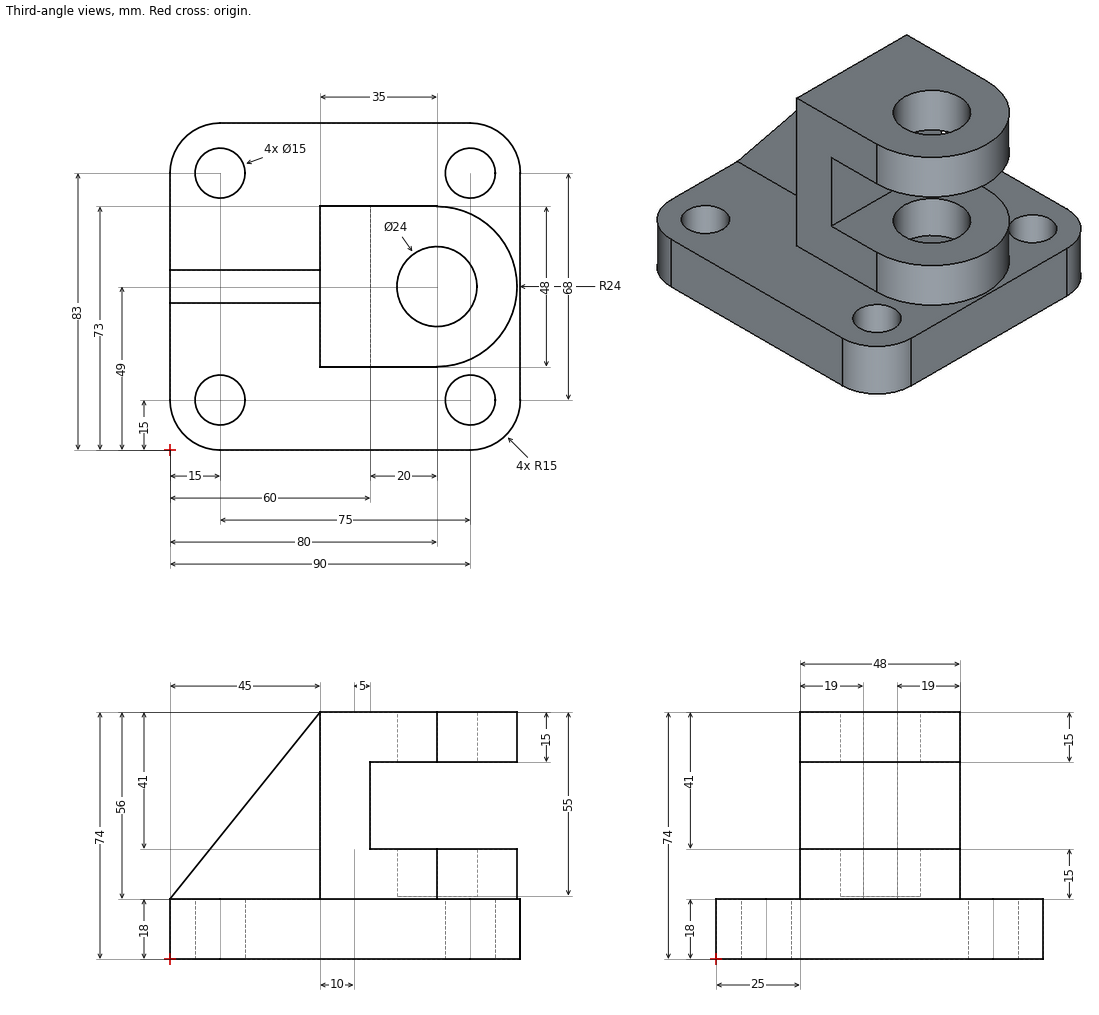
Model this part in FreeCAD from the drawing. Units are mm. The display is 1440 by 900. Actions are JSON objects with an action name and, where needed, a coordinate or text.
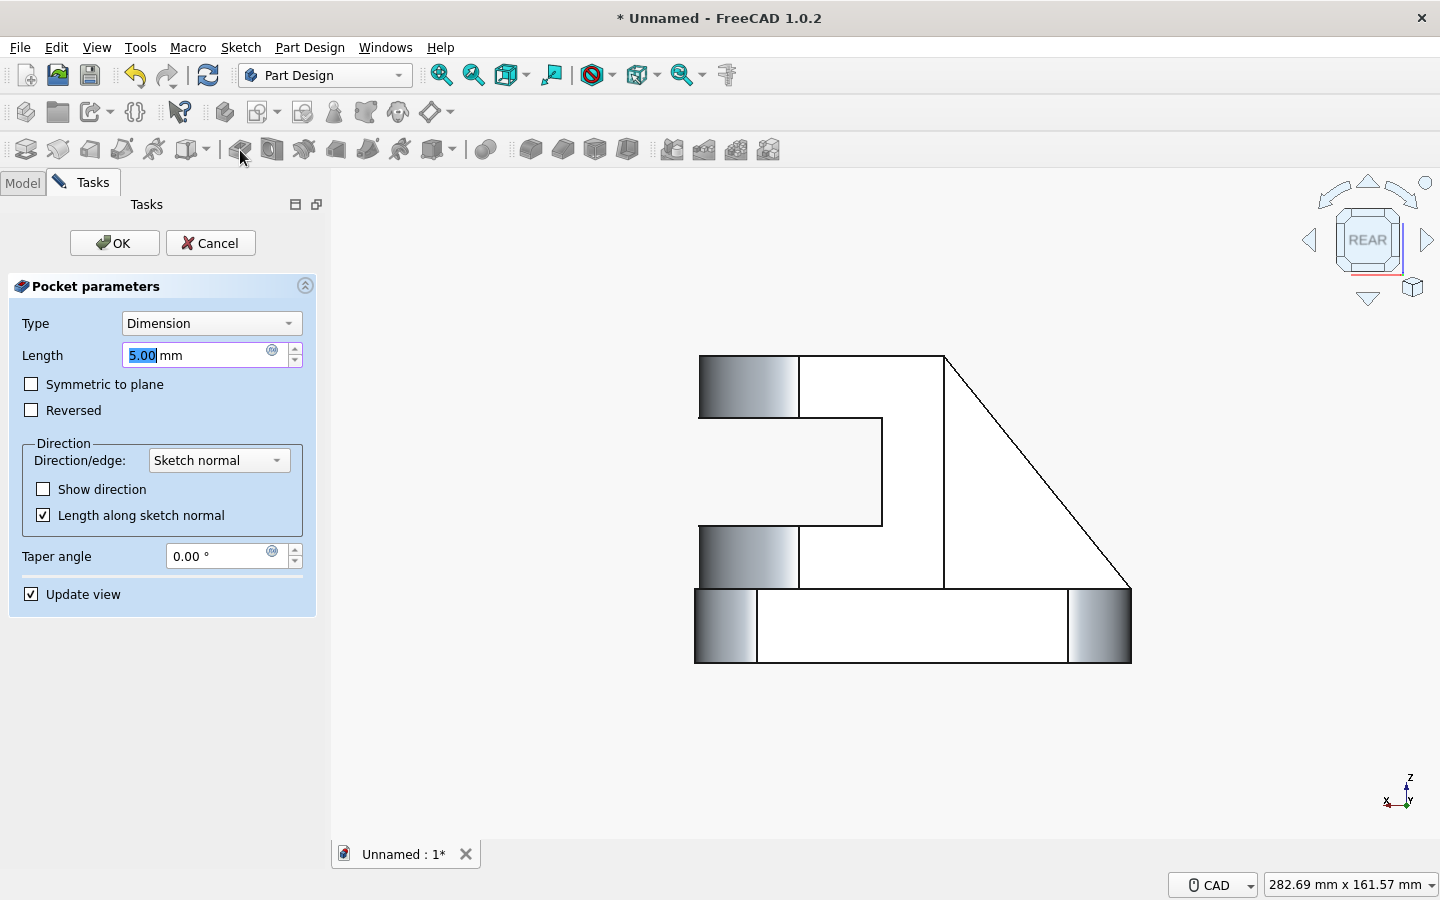
{"action": "type", "text": "19"}
{"action": "key", "text": "Tab"}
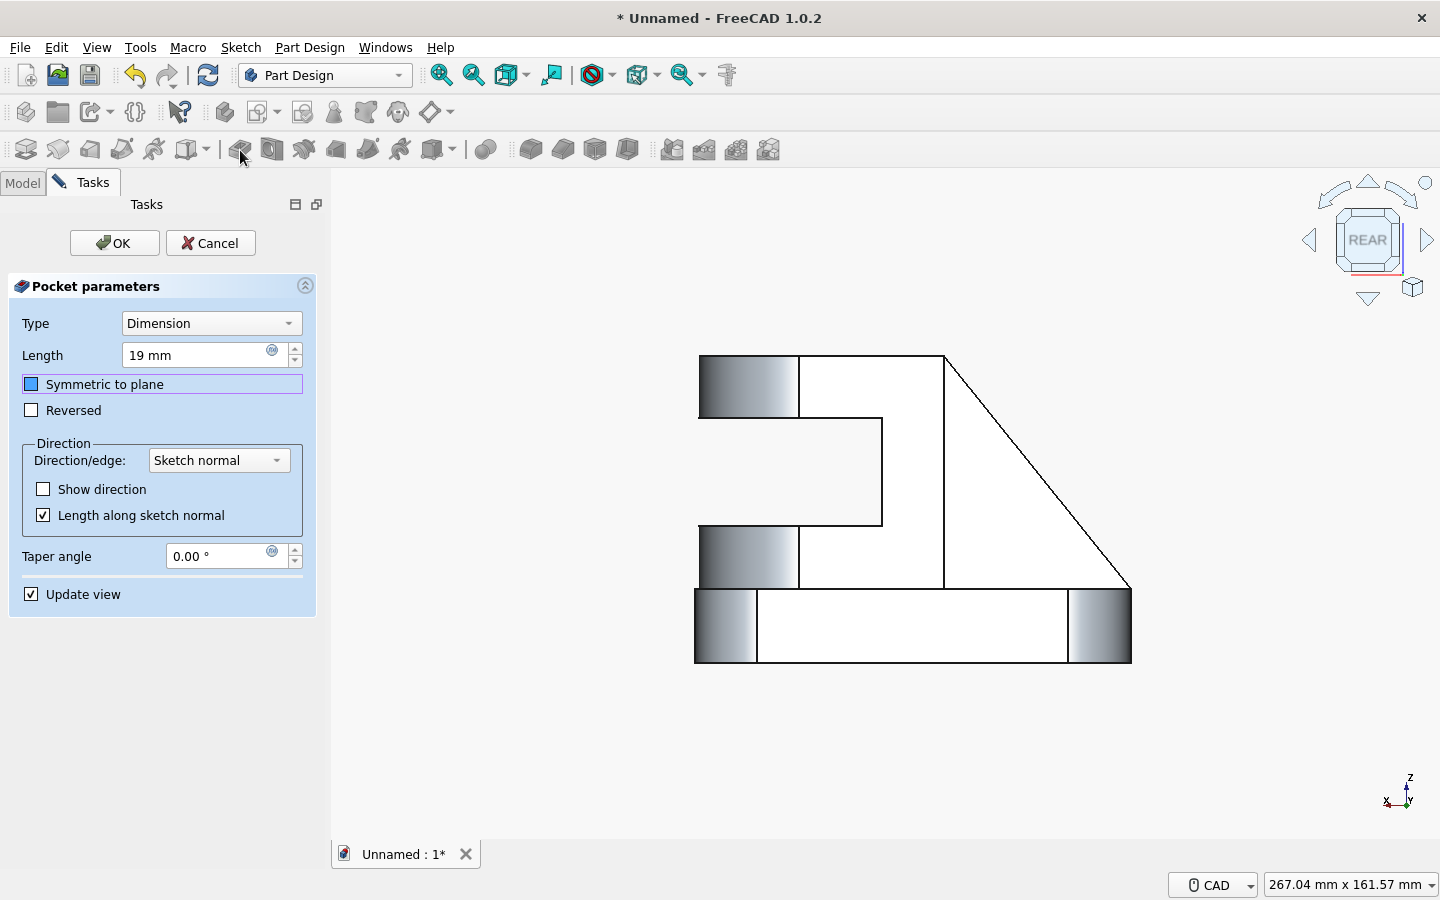
{"action": "left_click", "coordinate": [115, 243]}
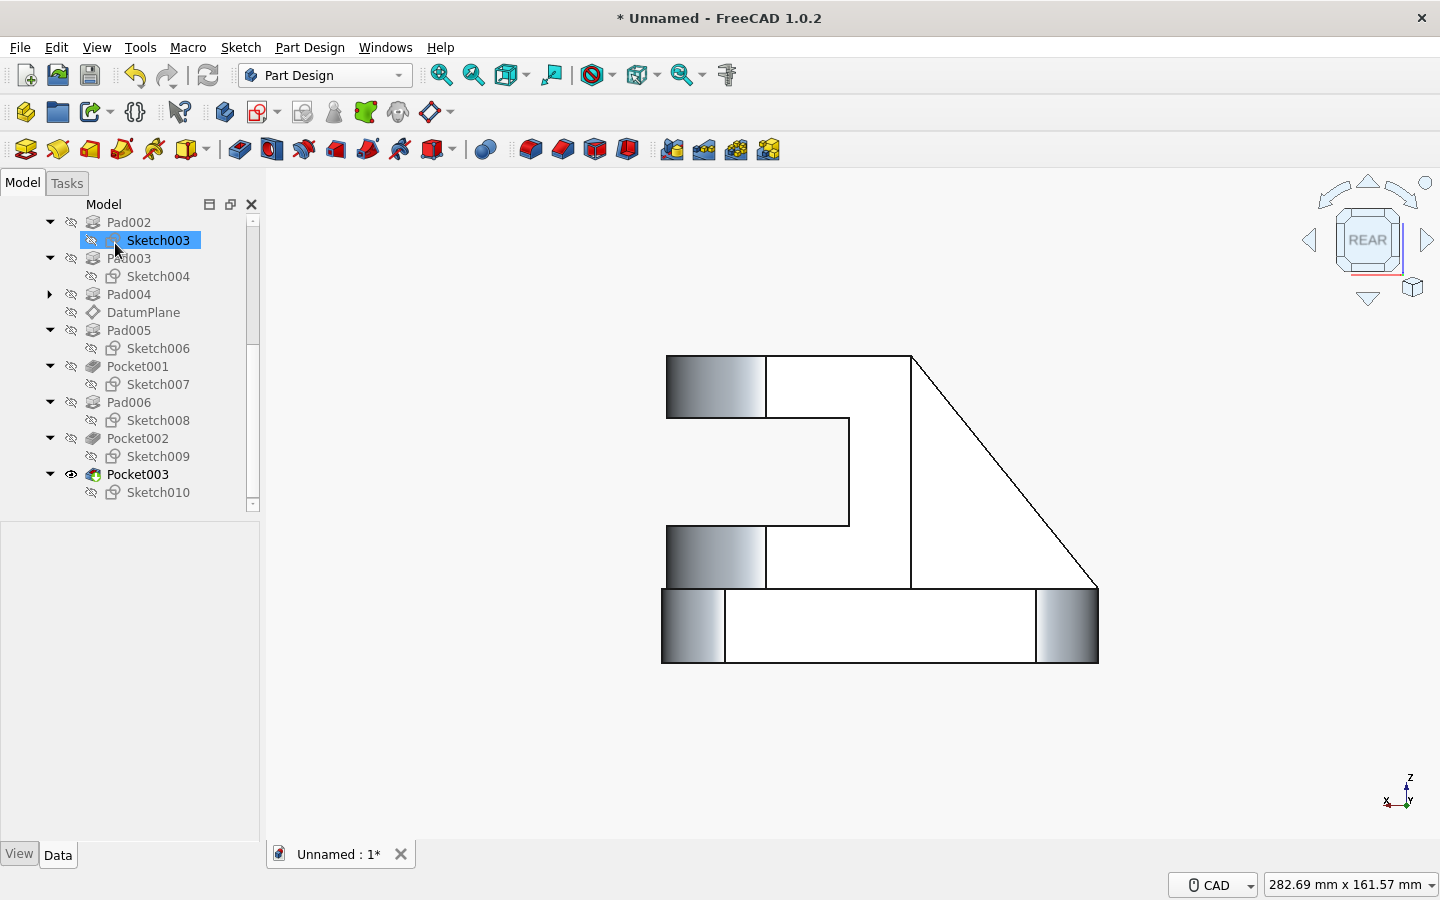
{"action": "key", "text": "0"}